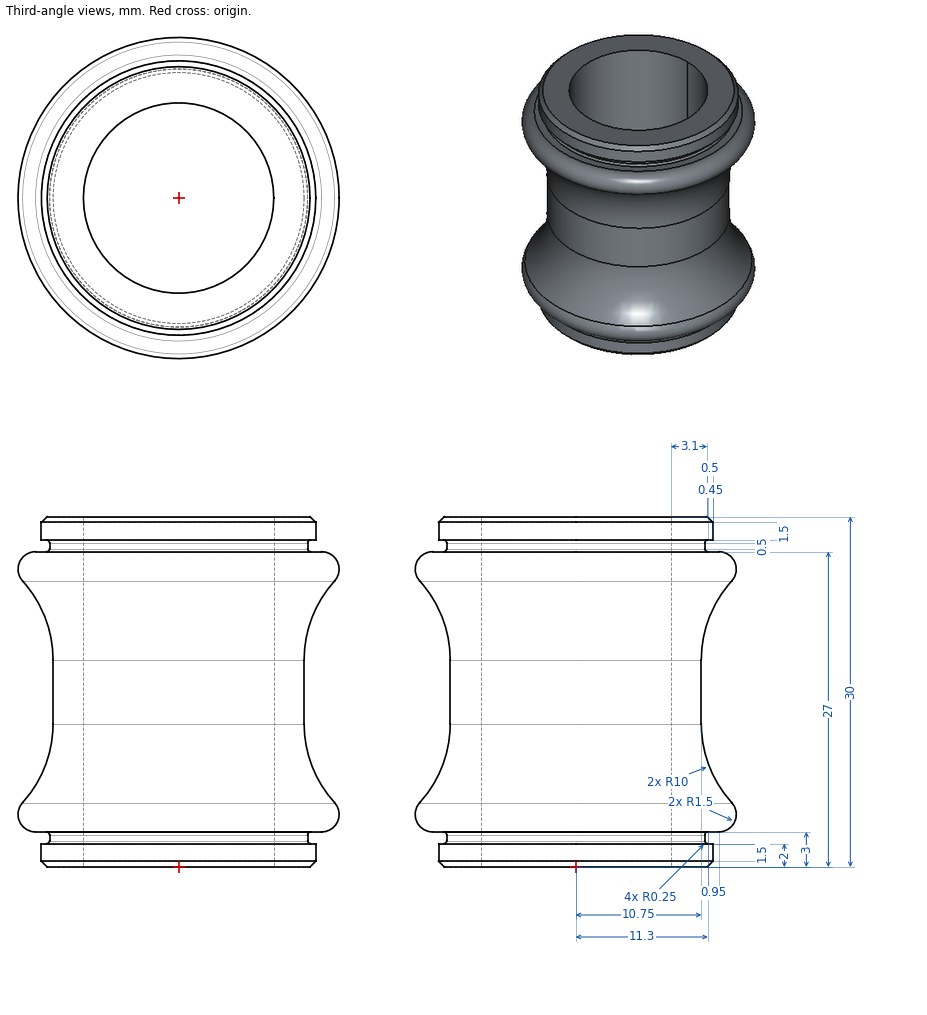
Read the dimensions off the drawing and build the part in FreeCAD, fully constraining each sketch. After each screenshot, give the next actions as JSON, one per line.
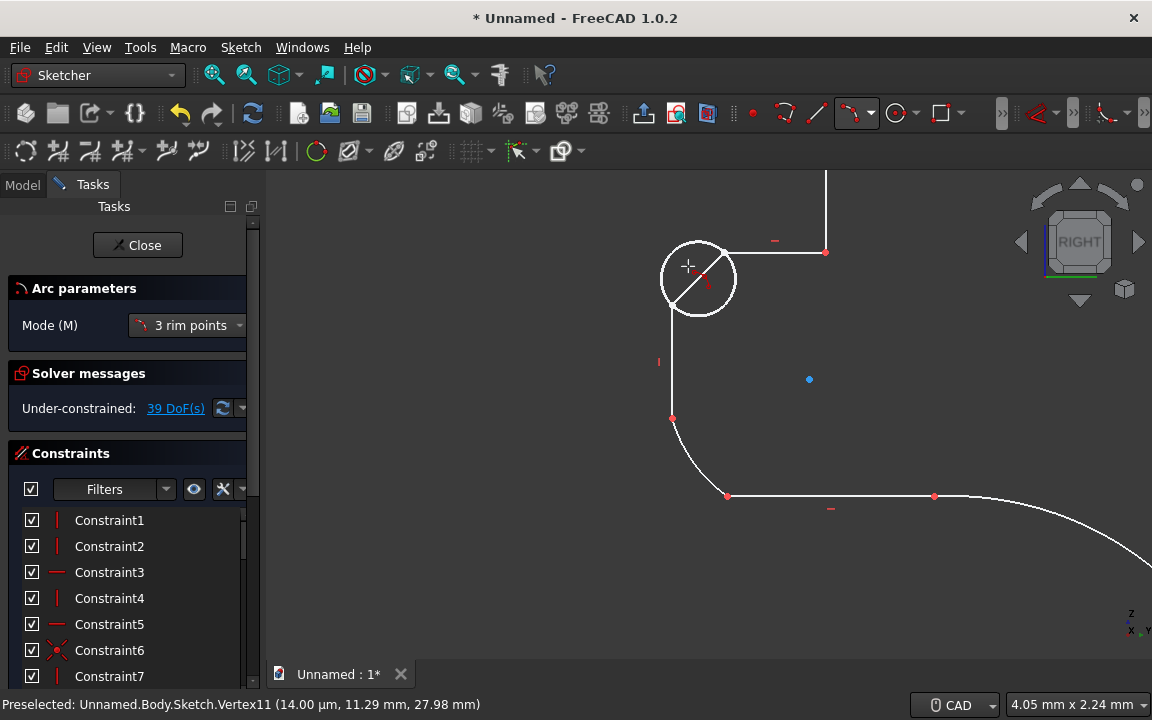
{"action": "left_click", "coordinate": [687, 264]}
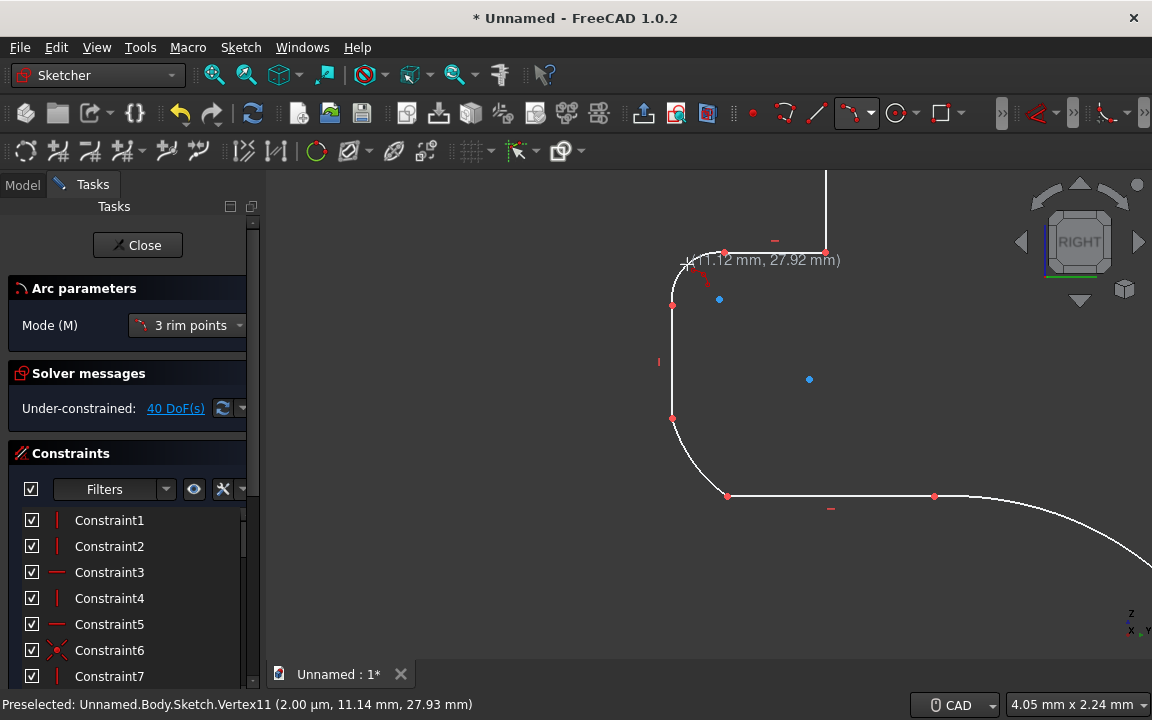
{"action": "scroll", "coordinate": [687, 274], "scroll_direction": "down", "scroll_amount": 15}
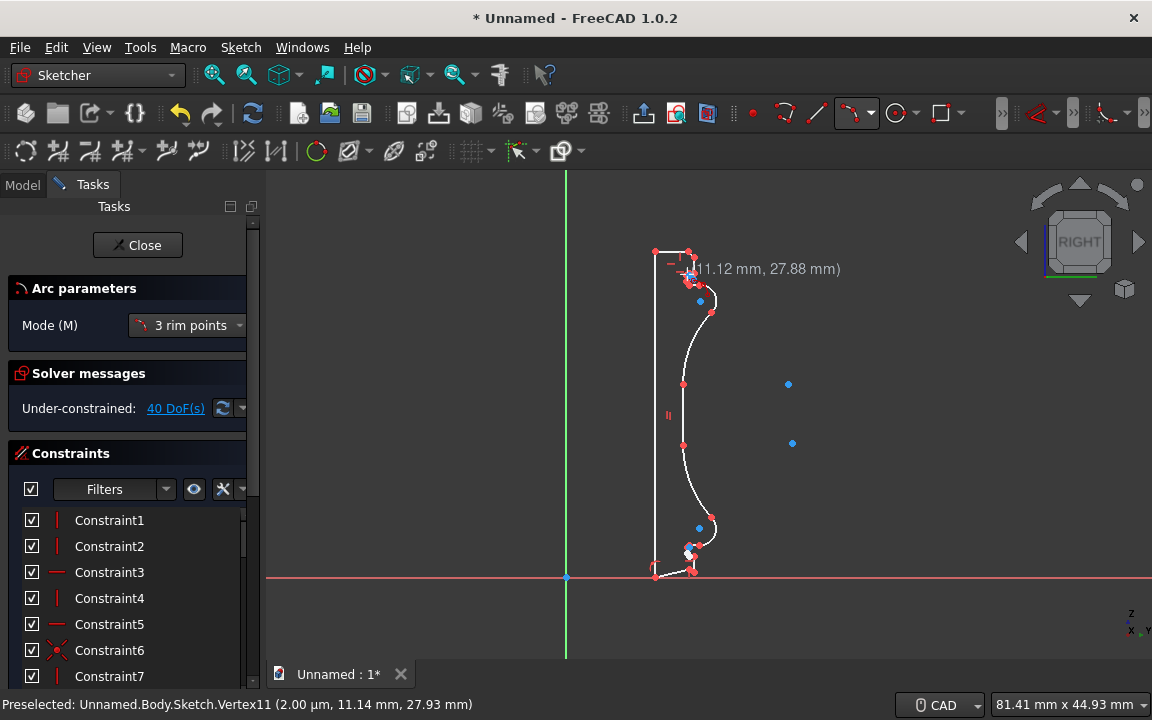
{"action": "scroll", "coordinate": [689, 556], "scroll_direction": "up", "scroll_amount": 10}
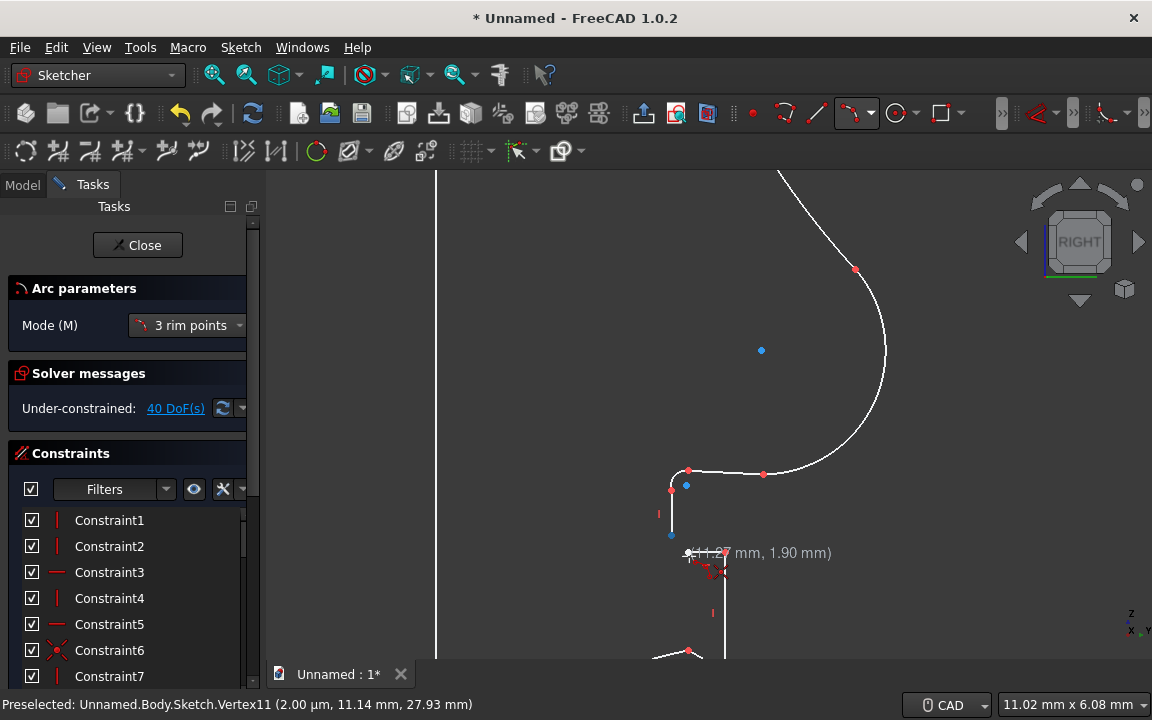
{"action": "left_click", "coordinate": [688, 552]}
{"action": "left_click", "coordinate": [672, 536]}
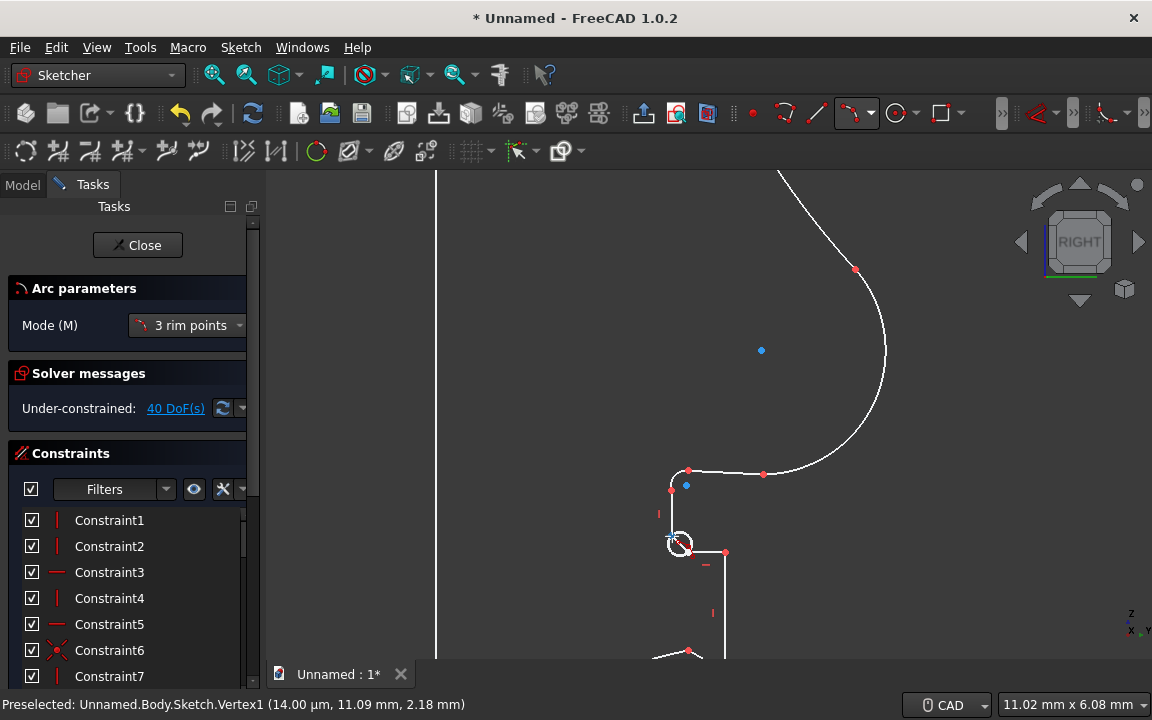
{"action": "scroll", "coordinate": [675, 544], "scroll_direction": "up", "scroll_amount": 5}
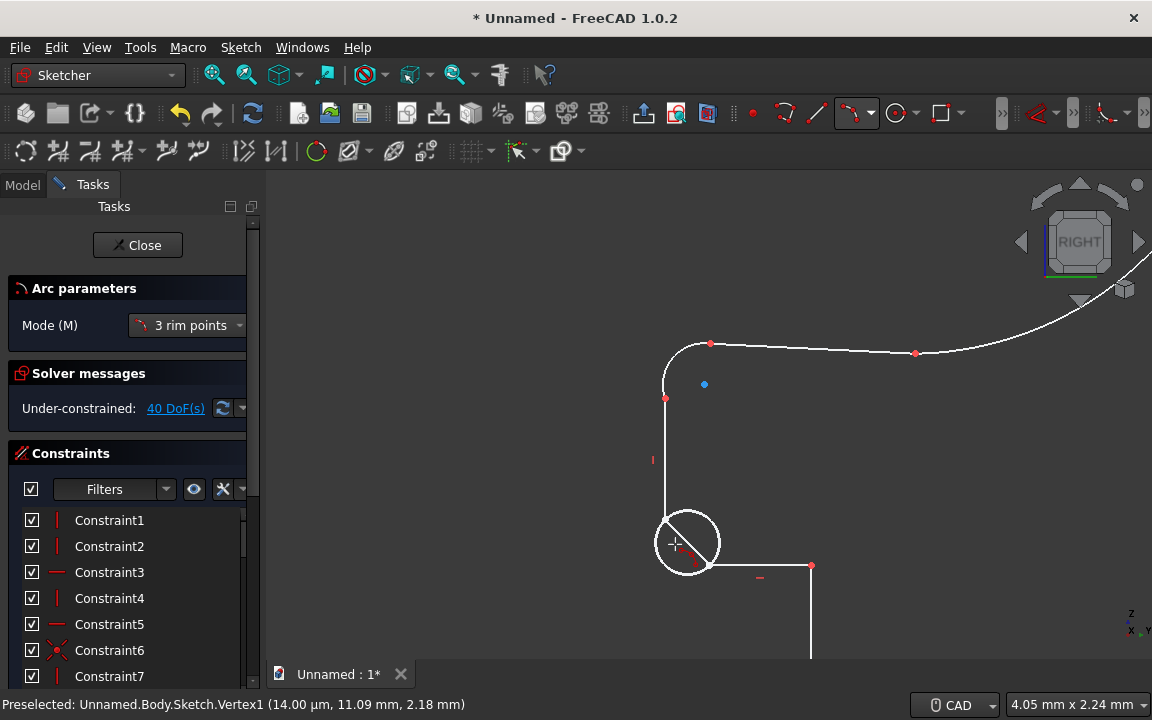
{"action": "left_click", "coordinate": [673, 543]}
{"action": "key", "text": "Escape"}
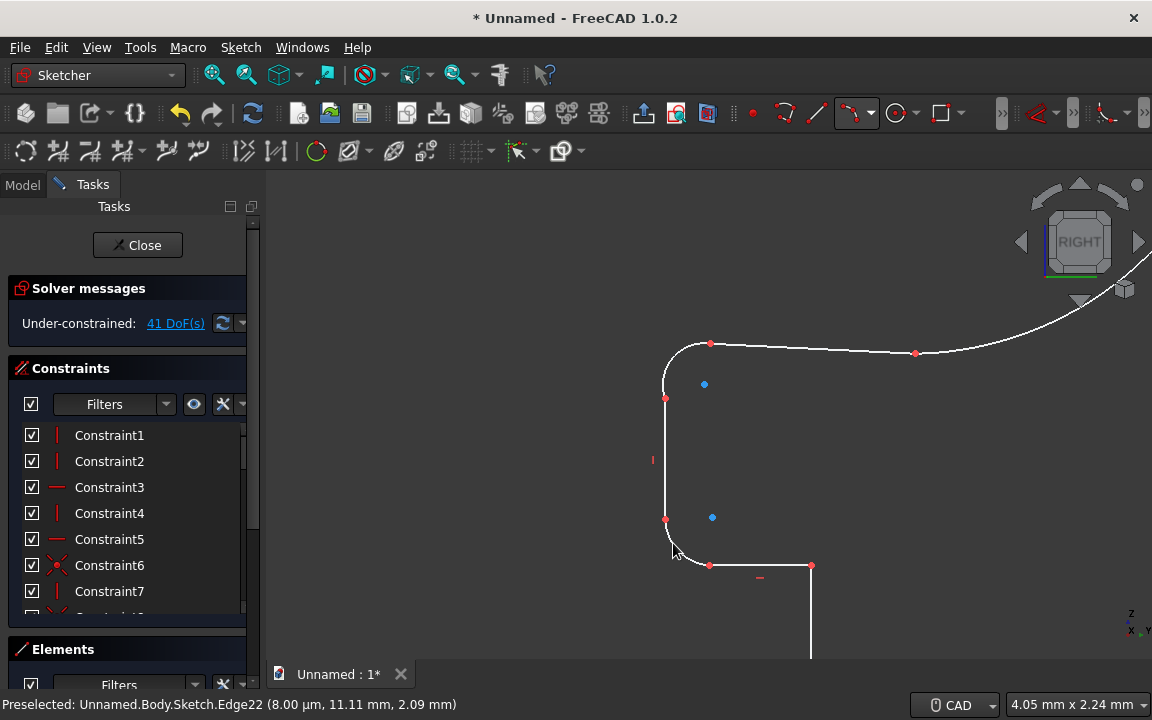
{"action": "left_click", "coordinate": [665, 483]}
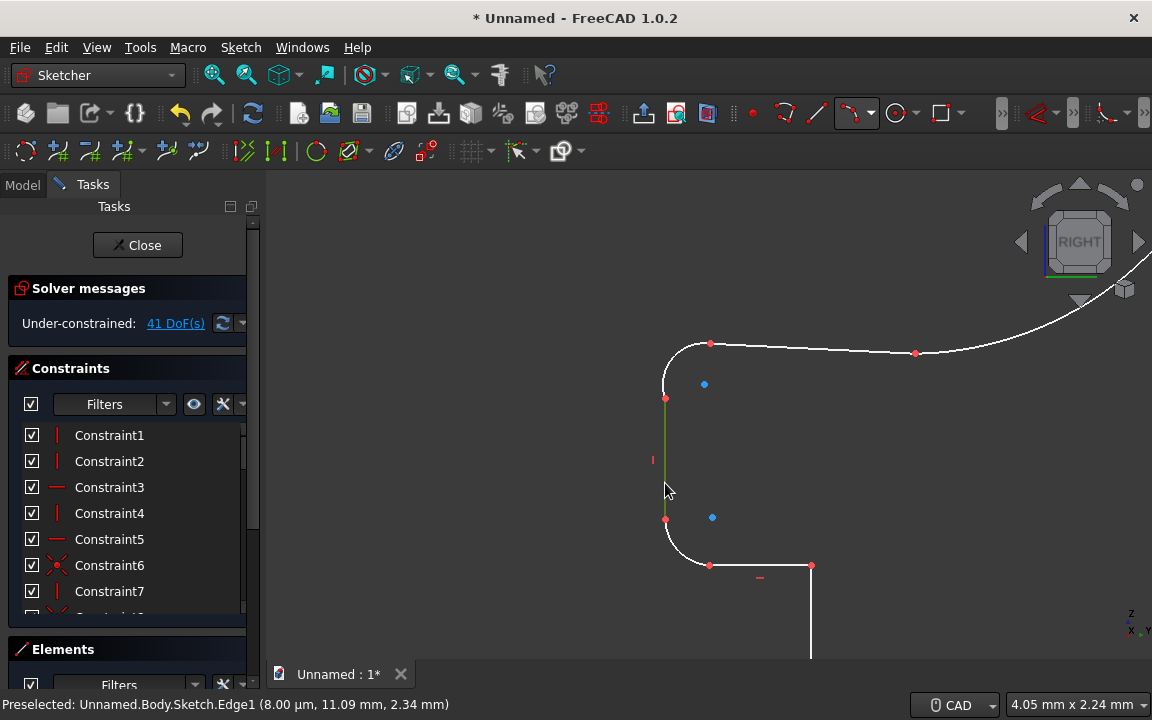
{"action": "left_click", "coordinate": [686, 348]}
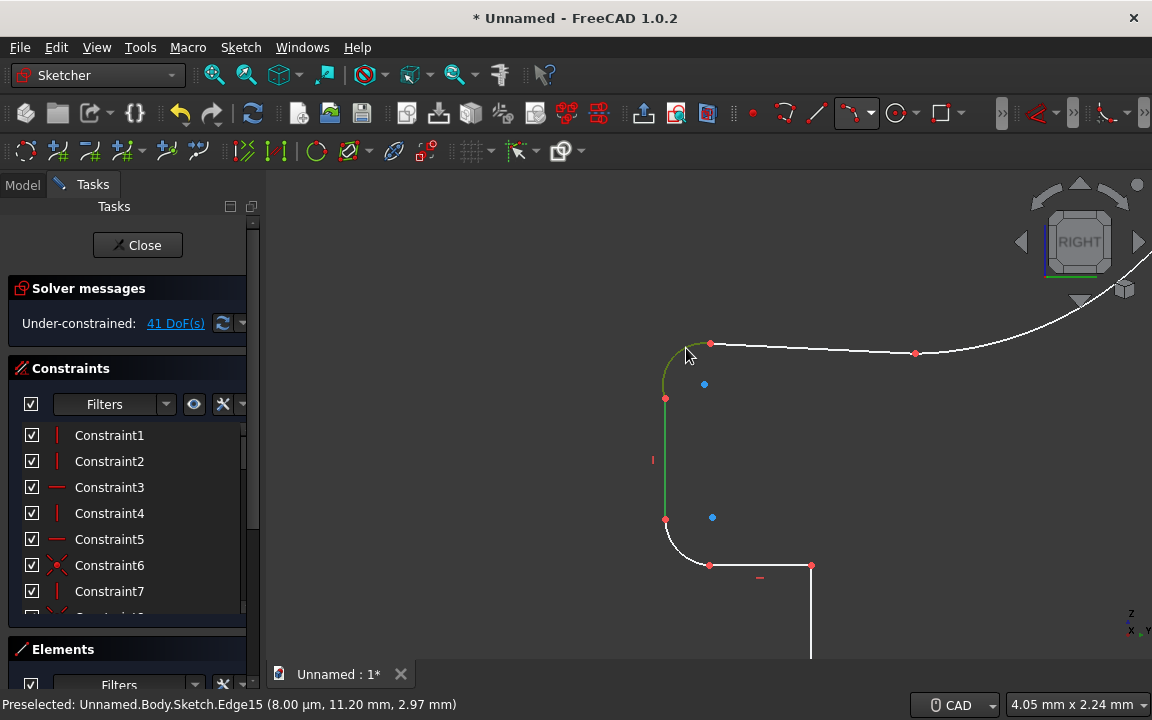
{"action": "key", "text": "t"}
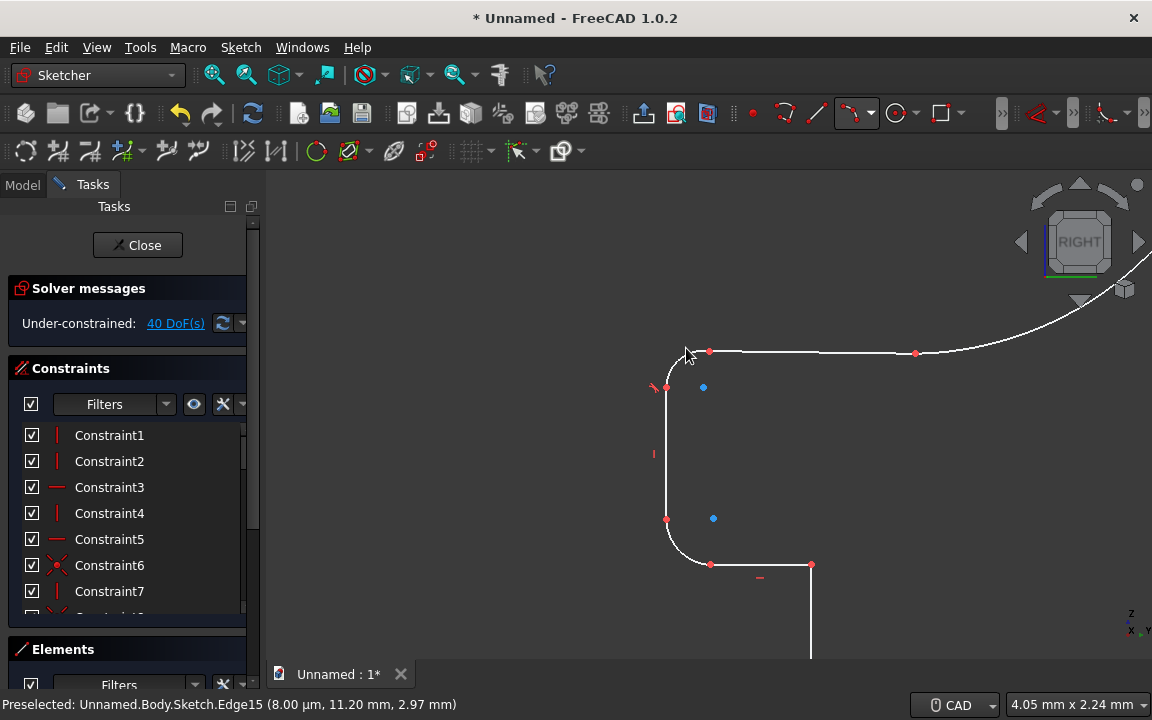
{"action": "scroll", "coordinate": [688, 556], "scroll_direction": "down", "scroll_amount": 15}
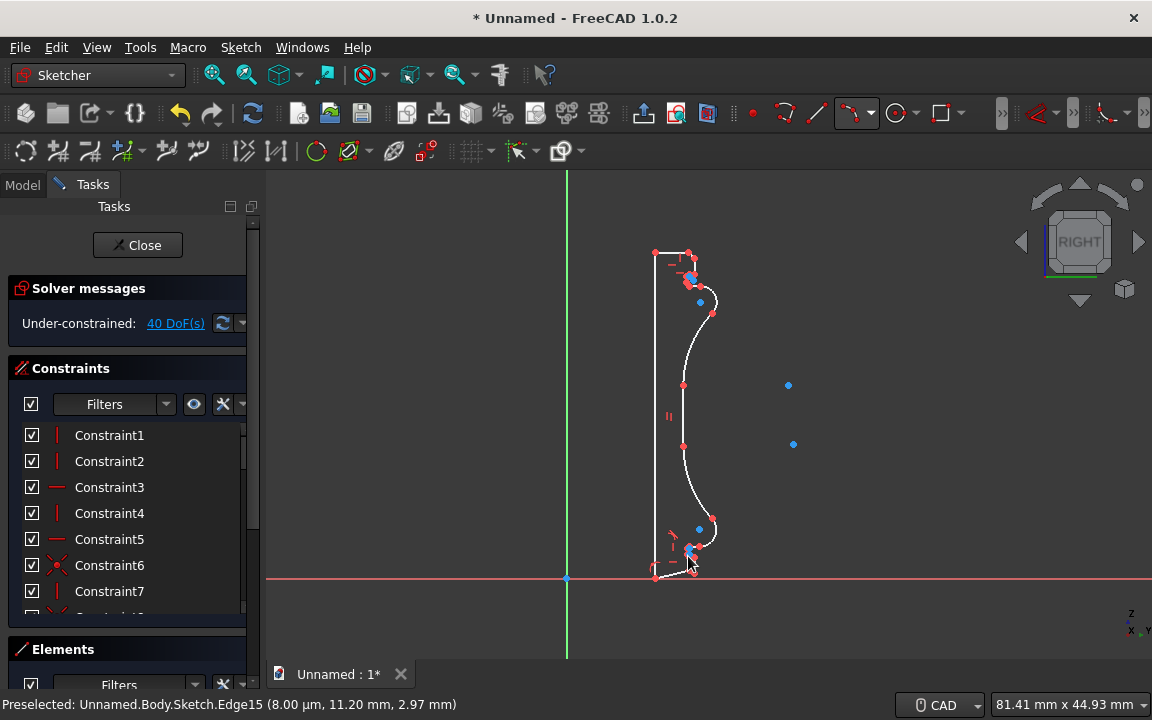
{"action": "scroll", "coordinate": [687, 553], "scroll_direction": "up", "scroll_amount": 10}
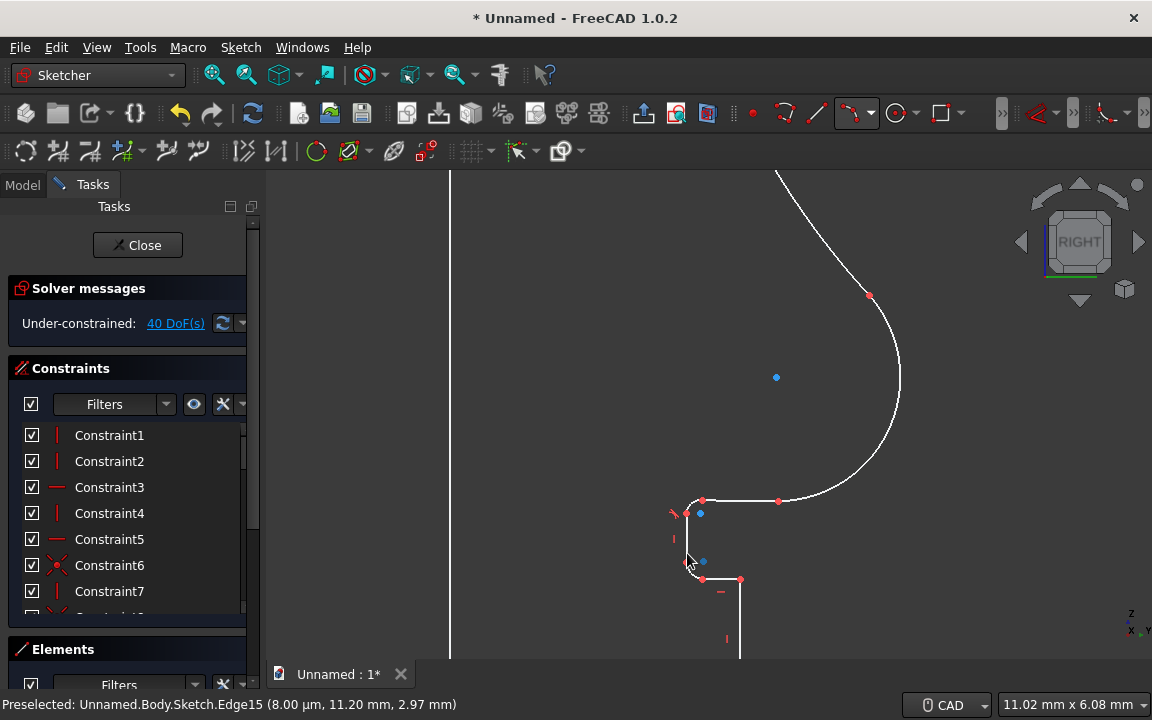
{"action": "left_click", "coordinate": [687, 548]}